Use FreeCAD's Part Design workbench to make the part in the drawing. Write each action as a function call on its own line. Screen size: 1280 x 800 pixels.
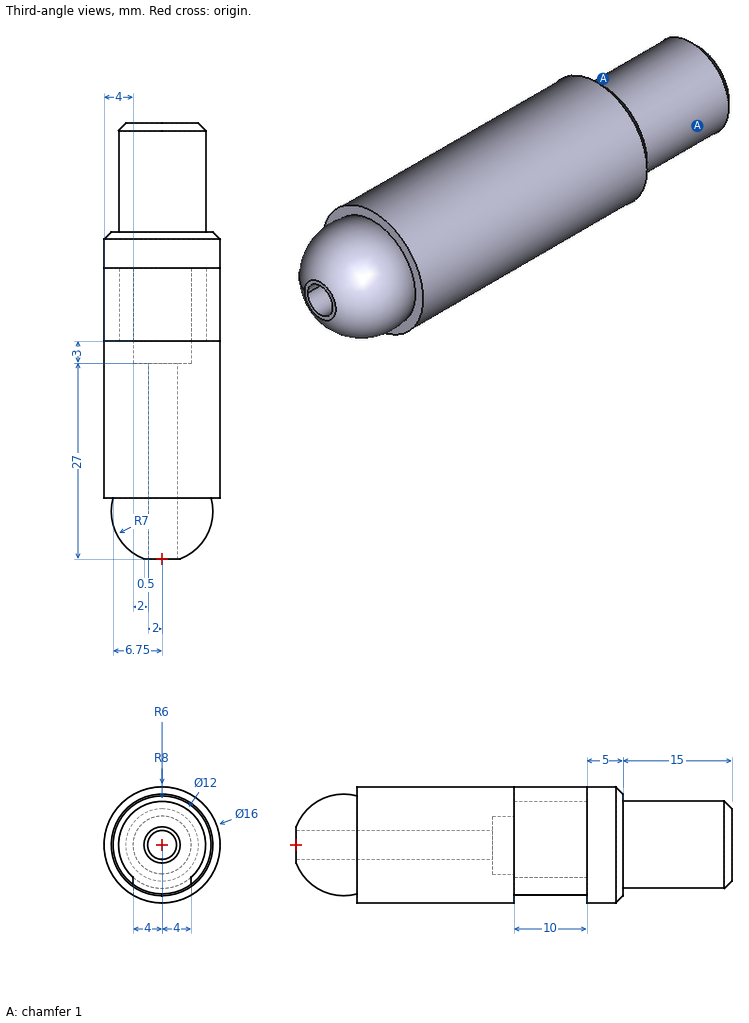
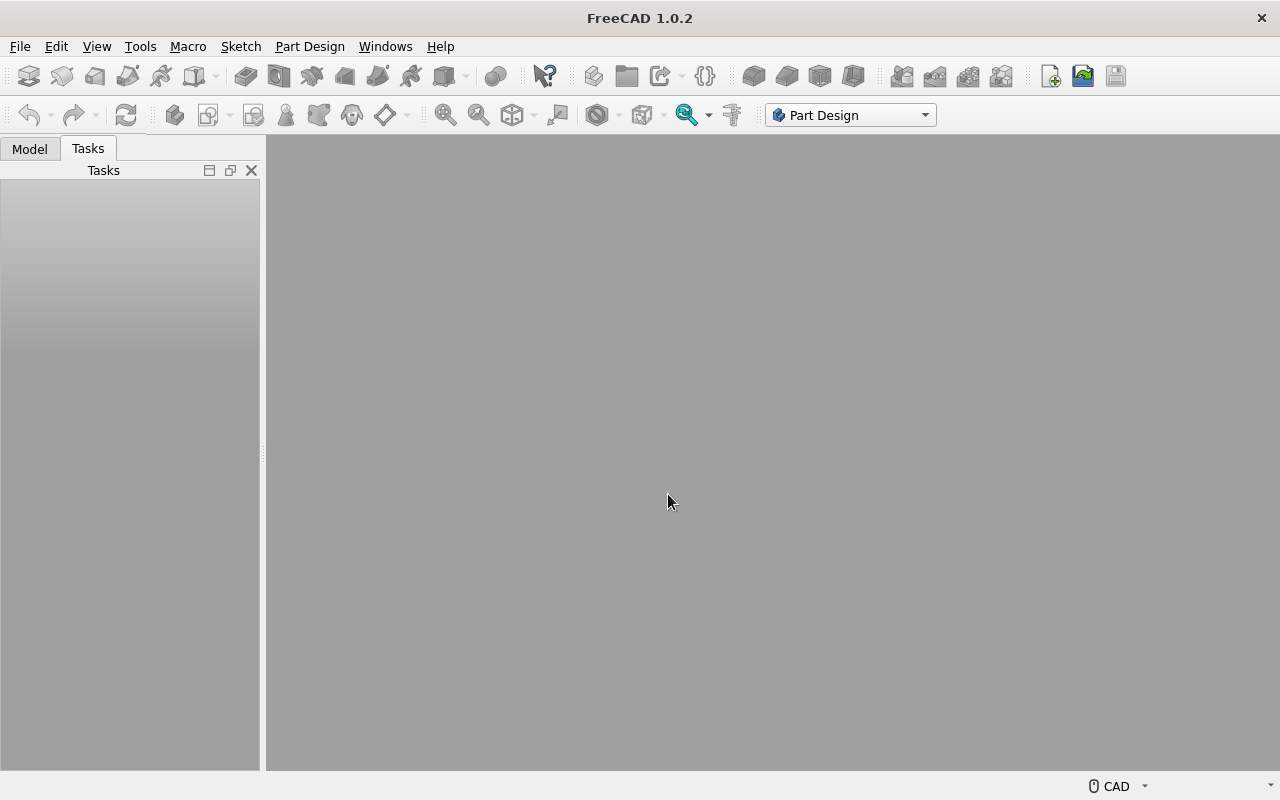
click(1050, 76)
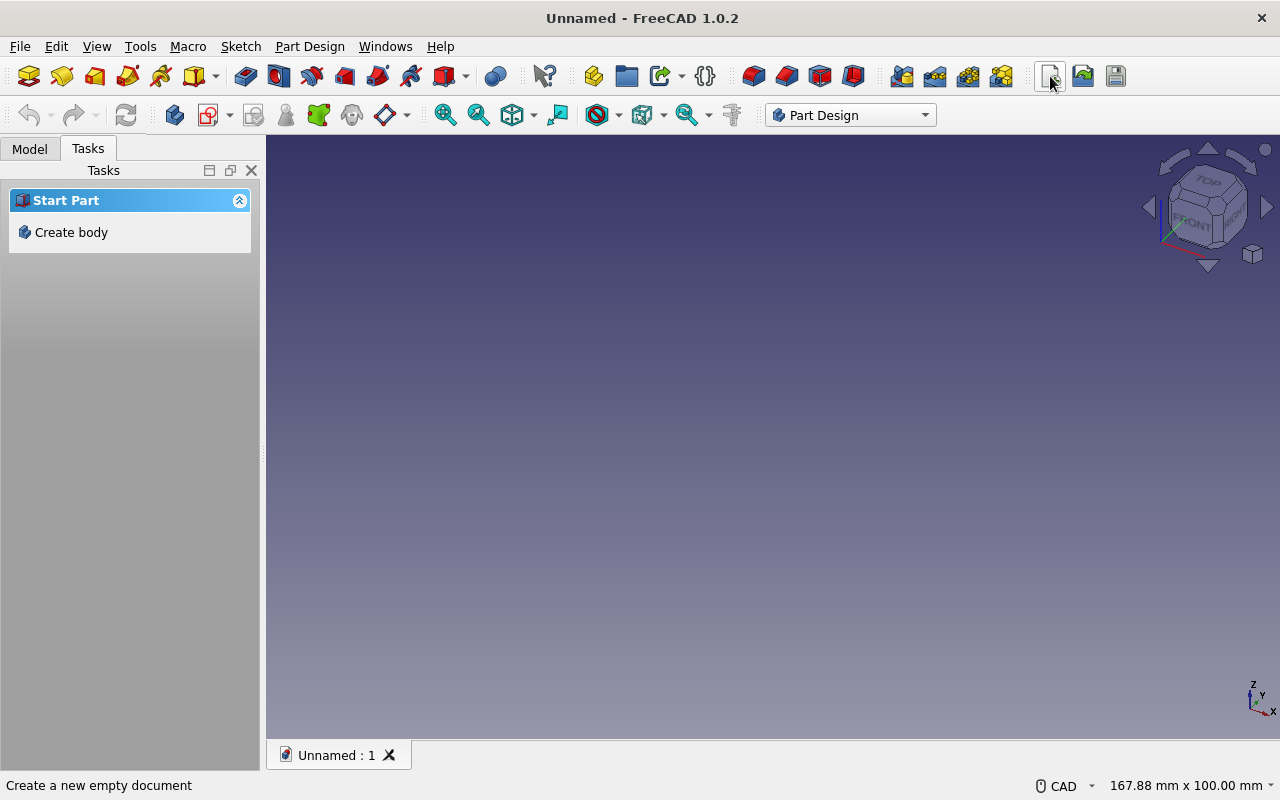
click(208, 116)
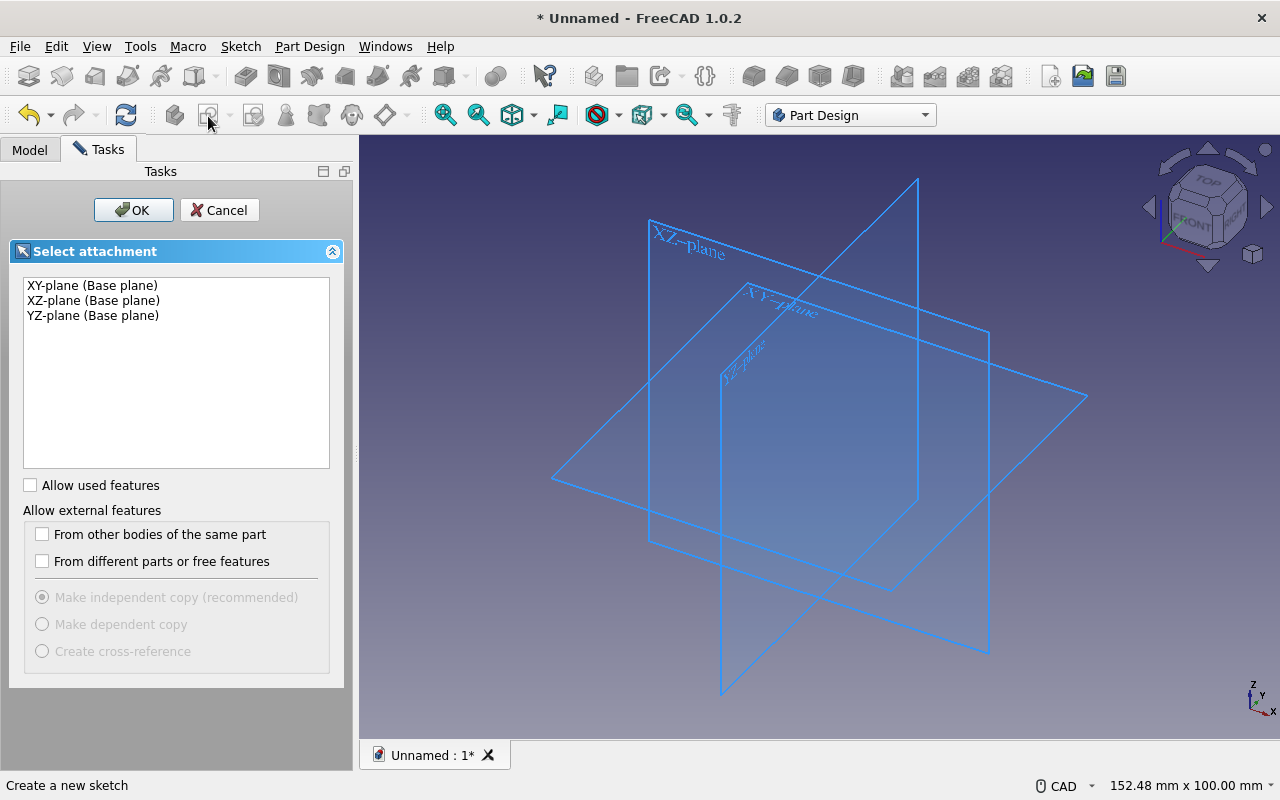
click(84, 286)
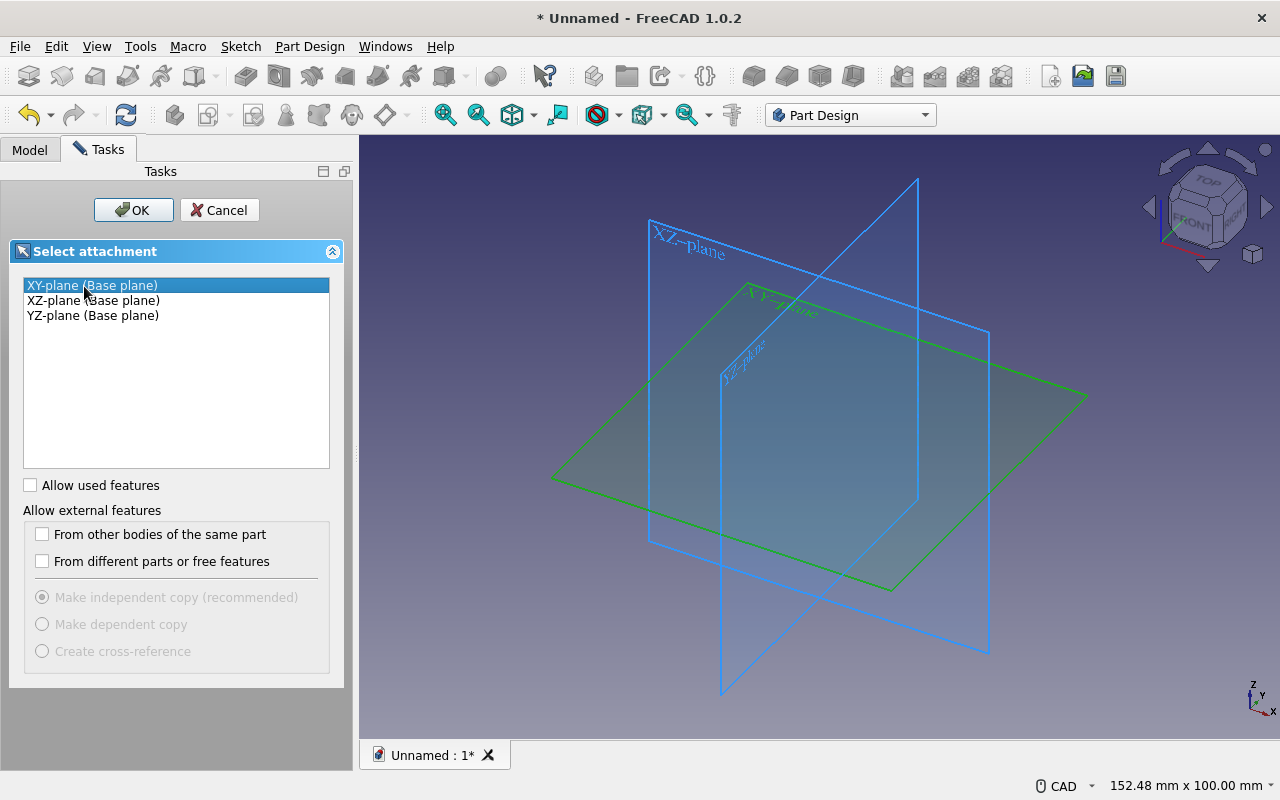
click(134, 210)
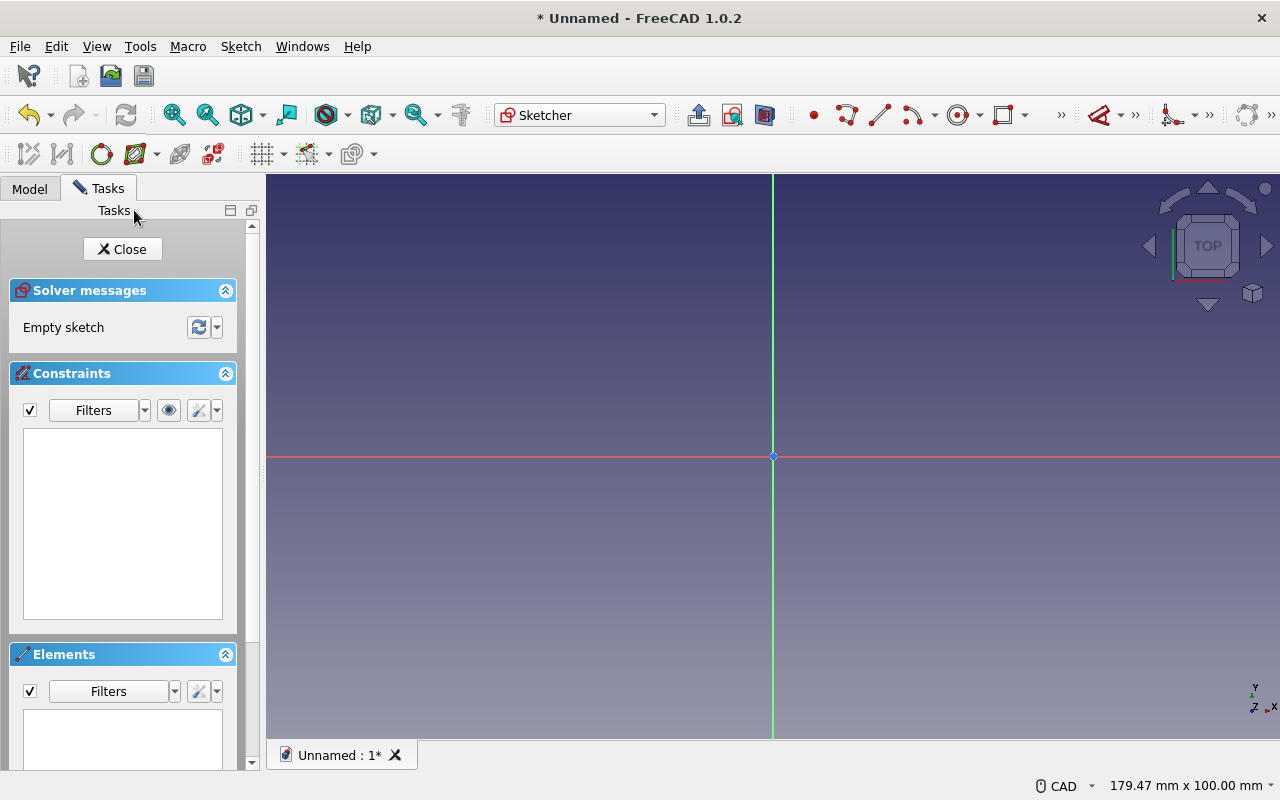
scroll(788, 303, up, 4)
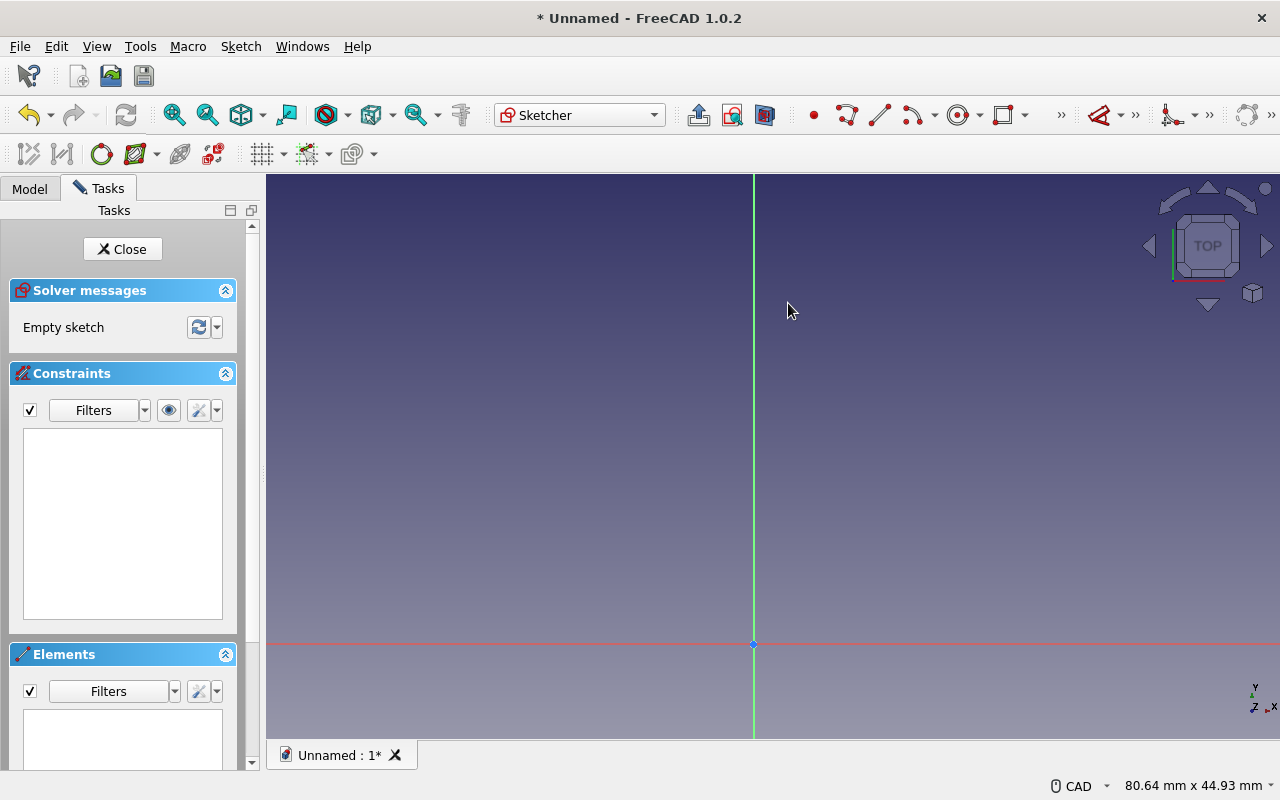
key(g)
key(m)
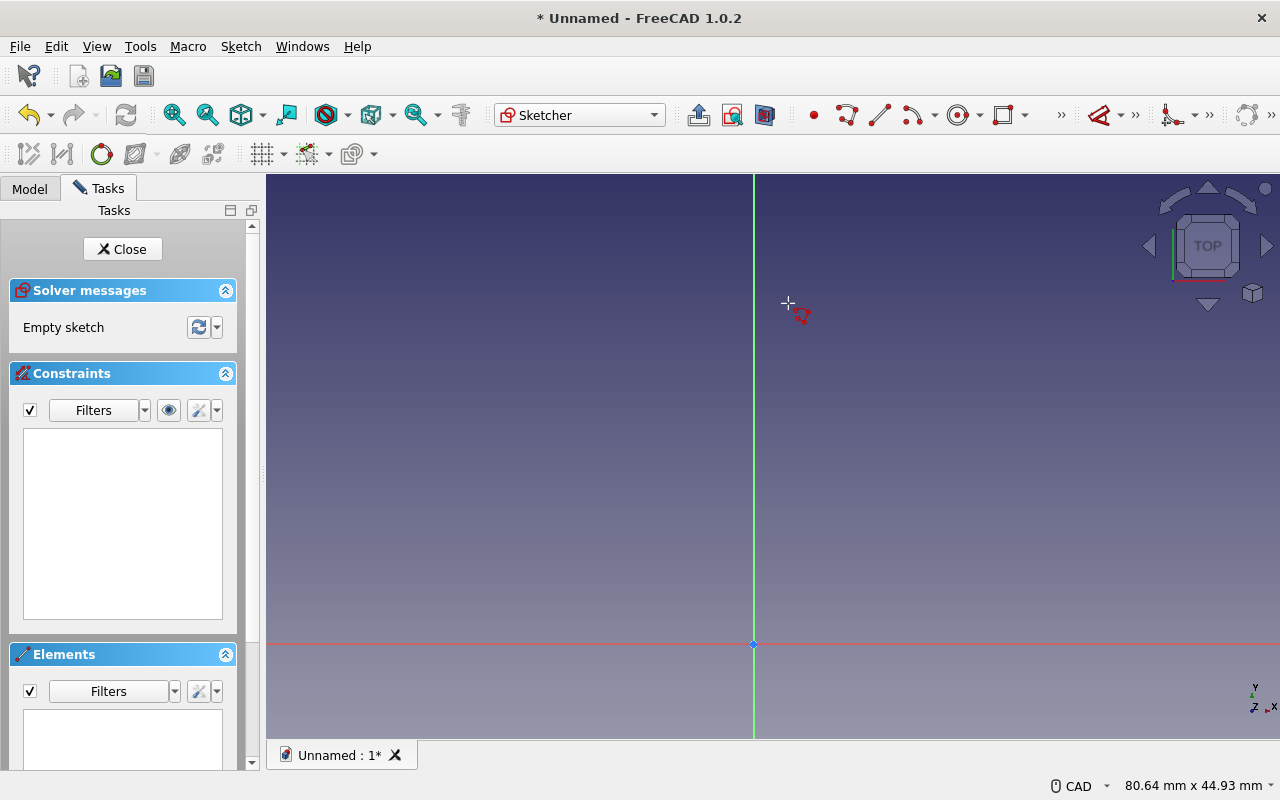
click(723, 644)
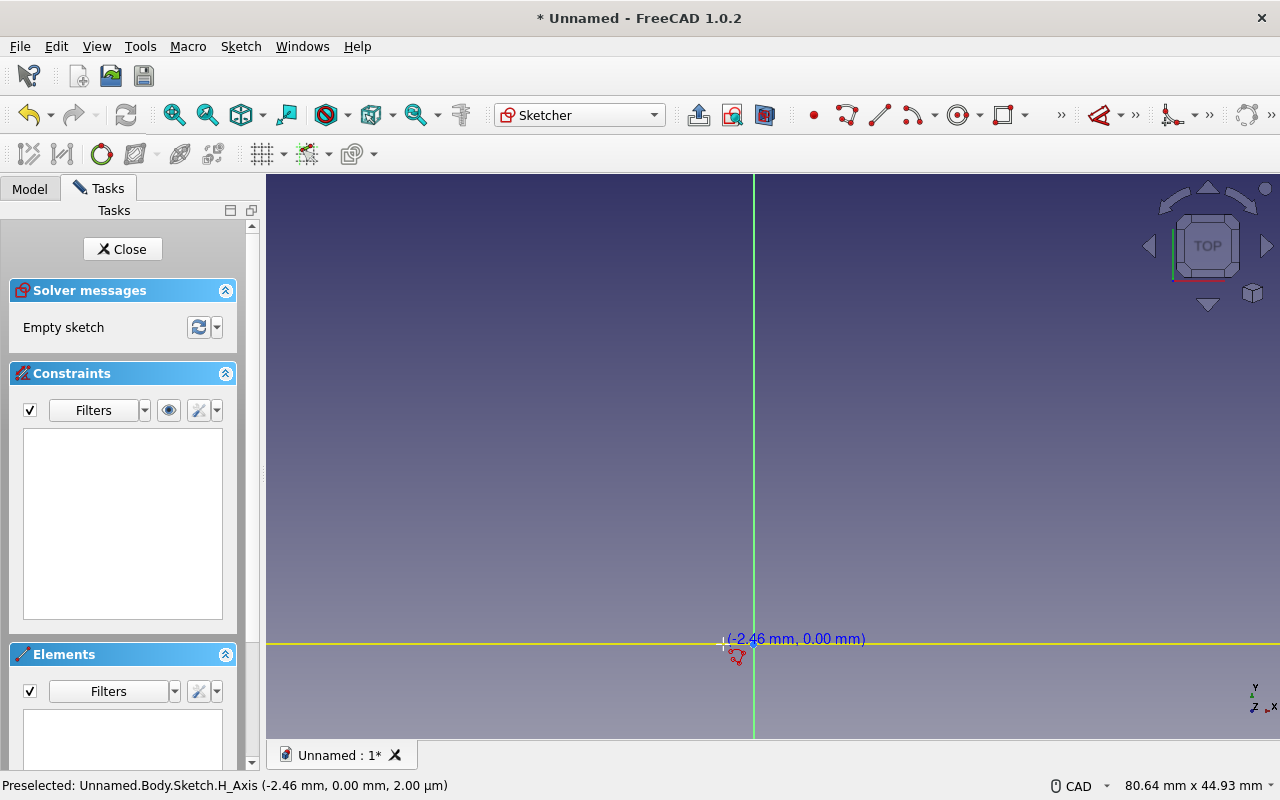
scroll(729, 644, up, 5)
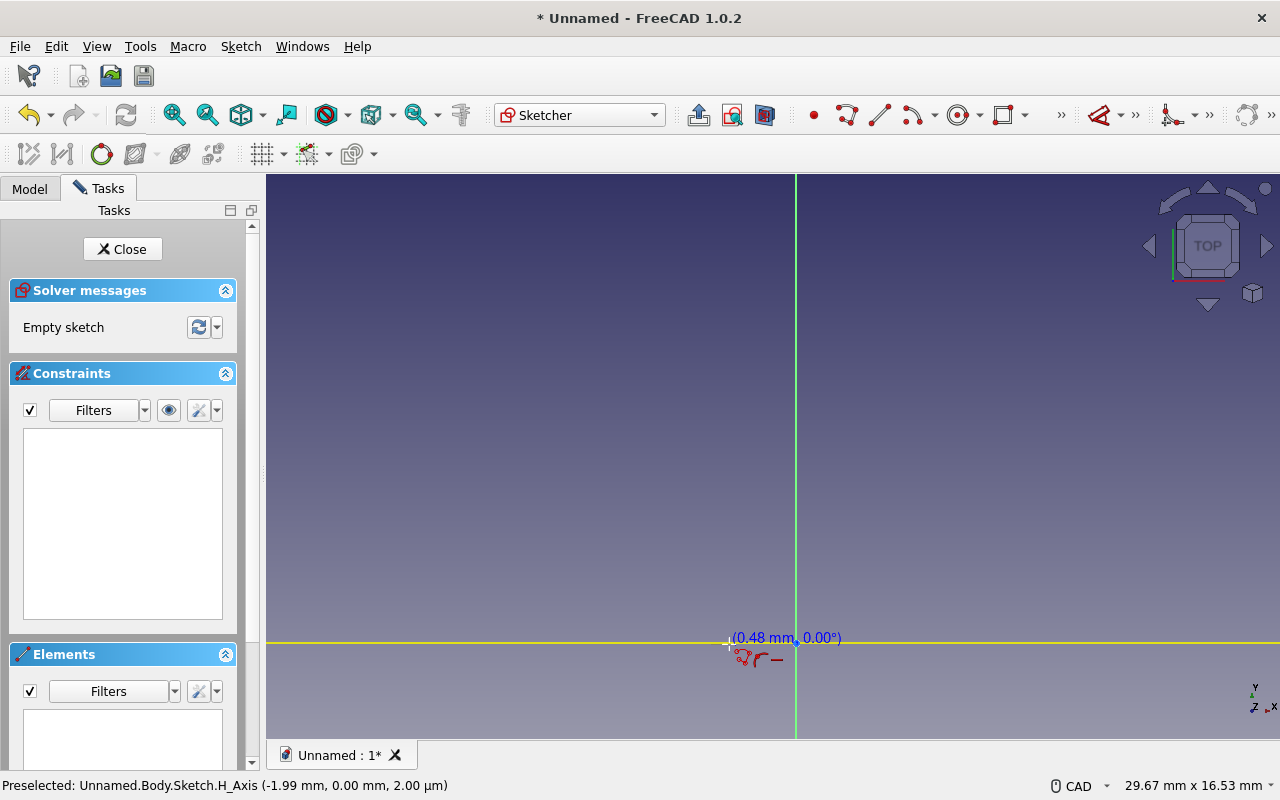
click(728, 634)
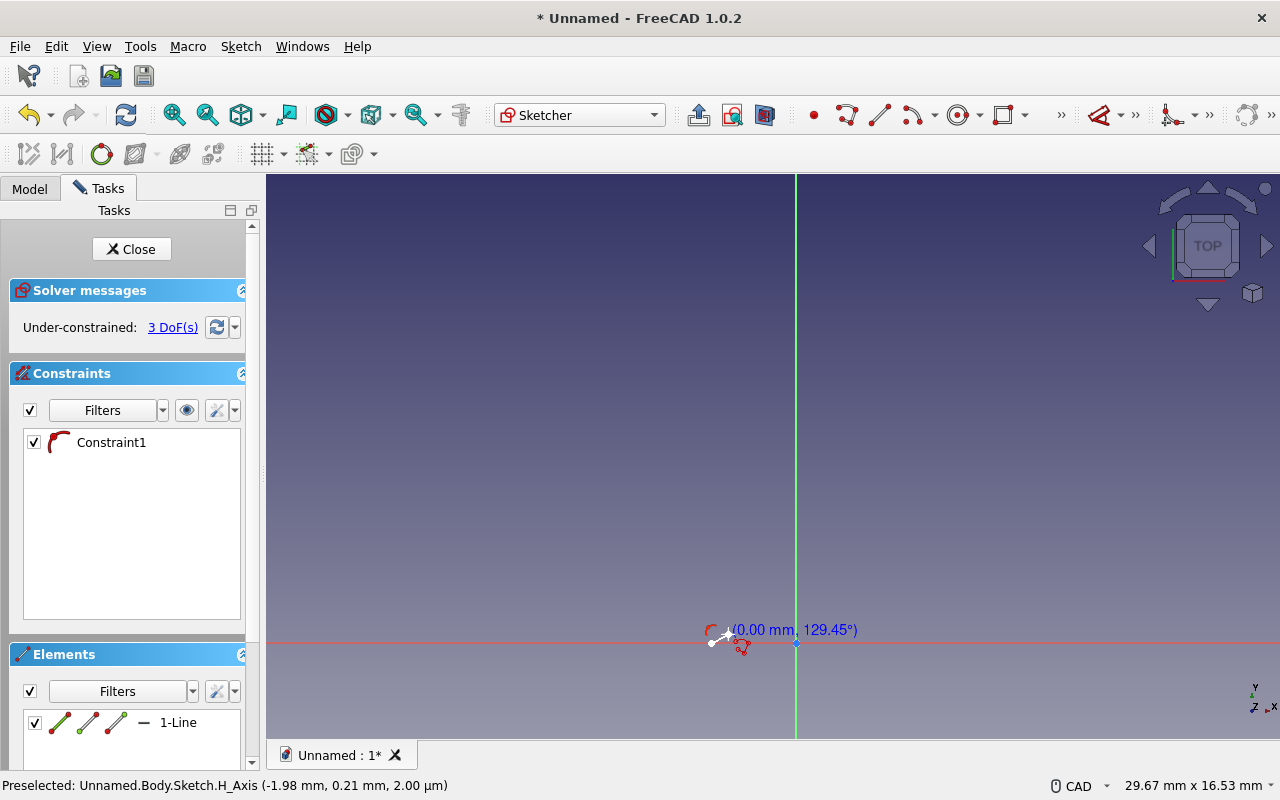
scroll(731, 646, down, 5)